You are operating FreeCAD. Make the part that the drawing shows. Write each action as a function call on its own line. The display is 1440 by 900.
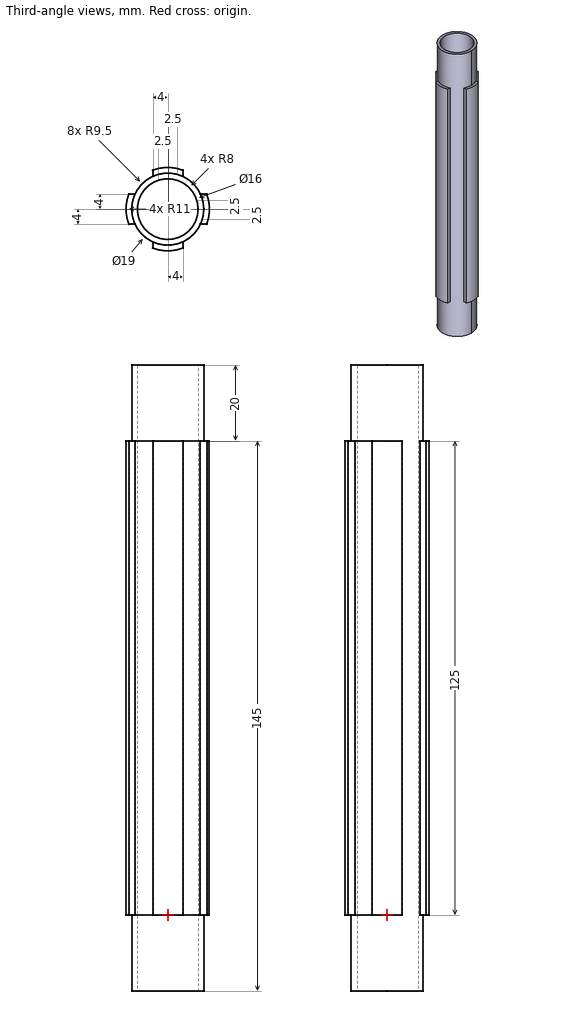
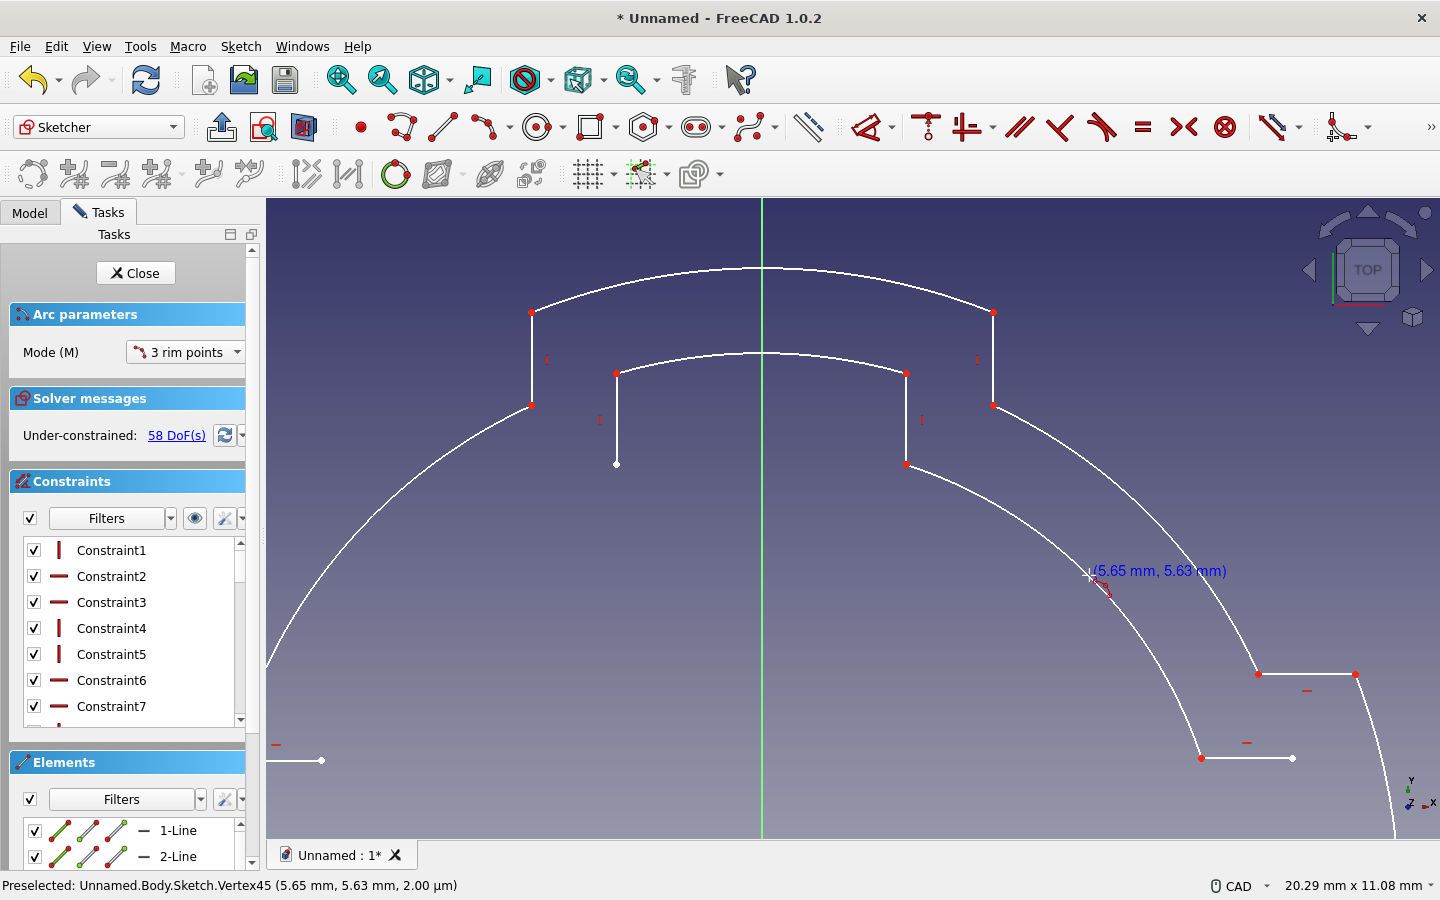
scroll(794, 353, down, 6)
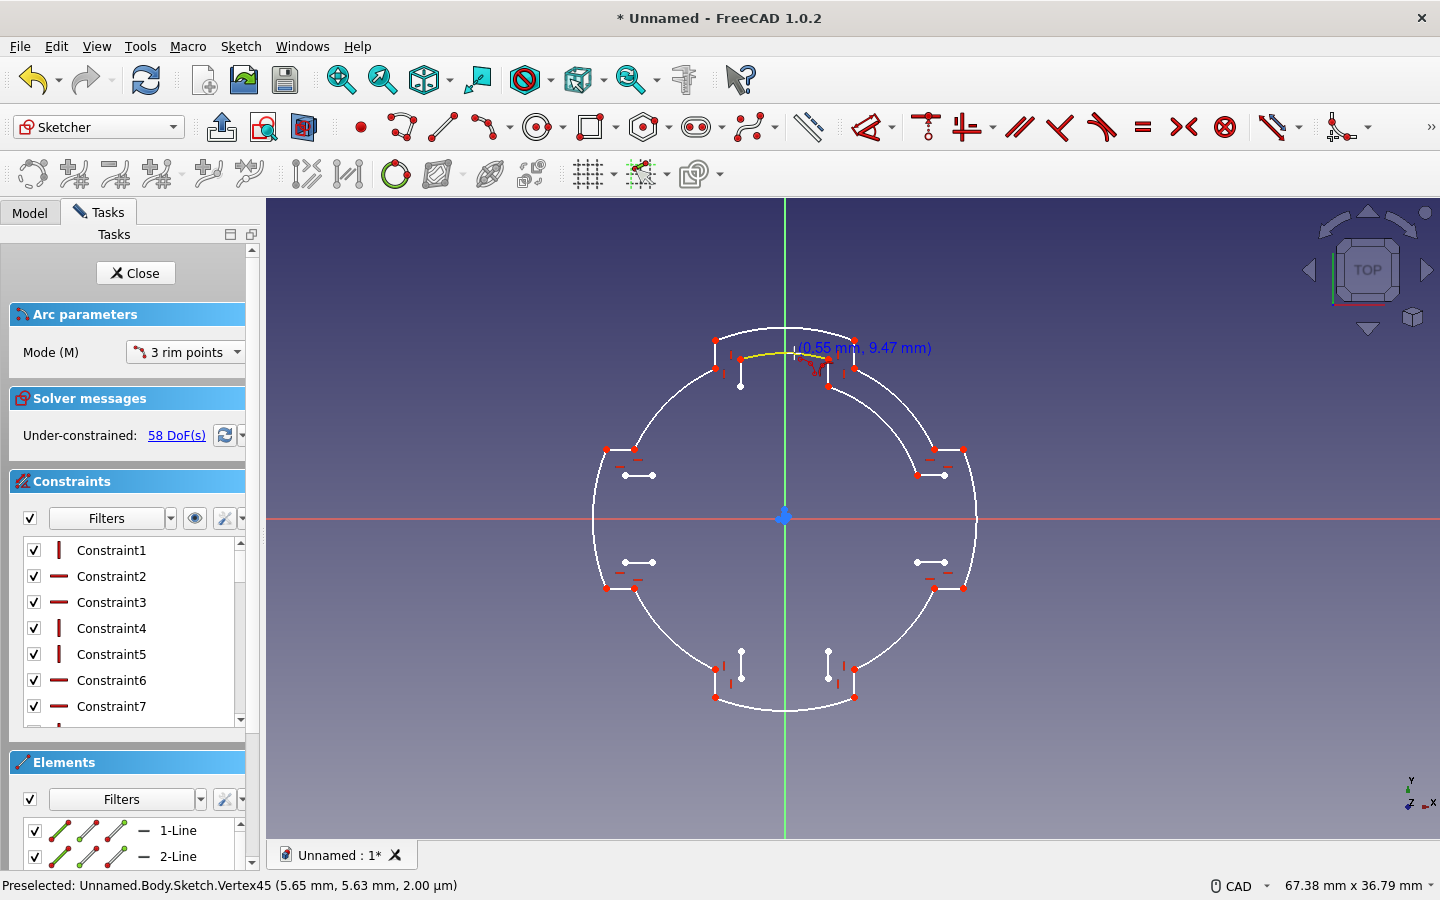
click(945, 475)
click(945, 562)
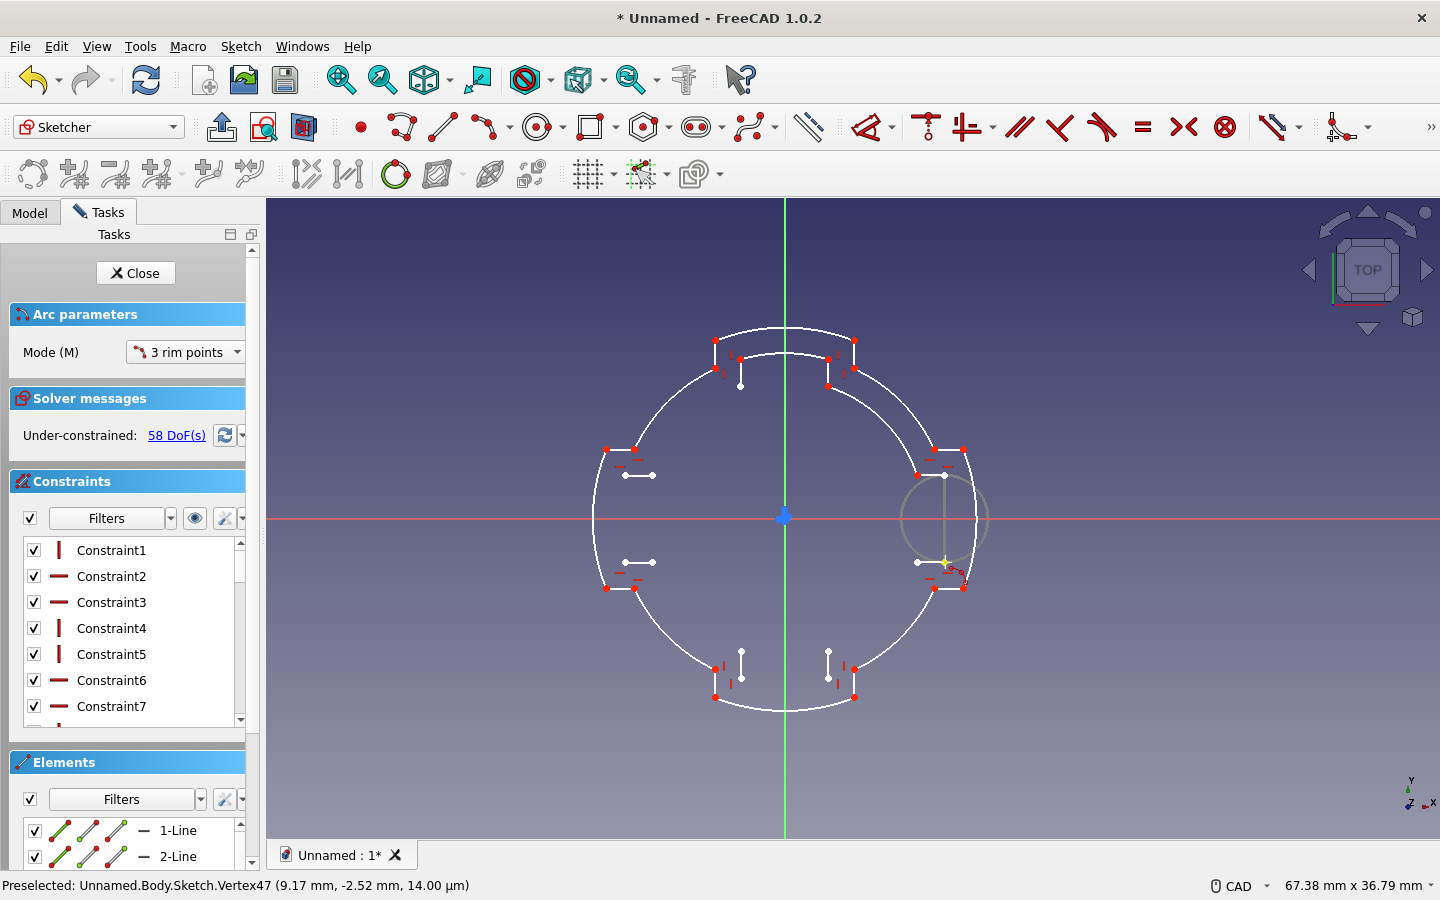
scroll(950, 527, up, 6)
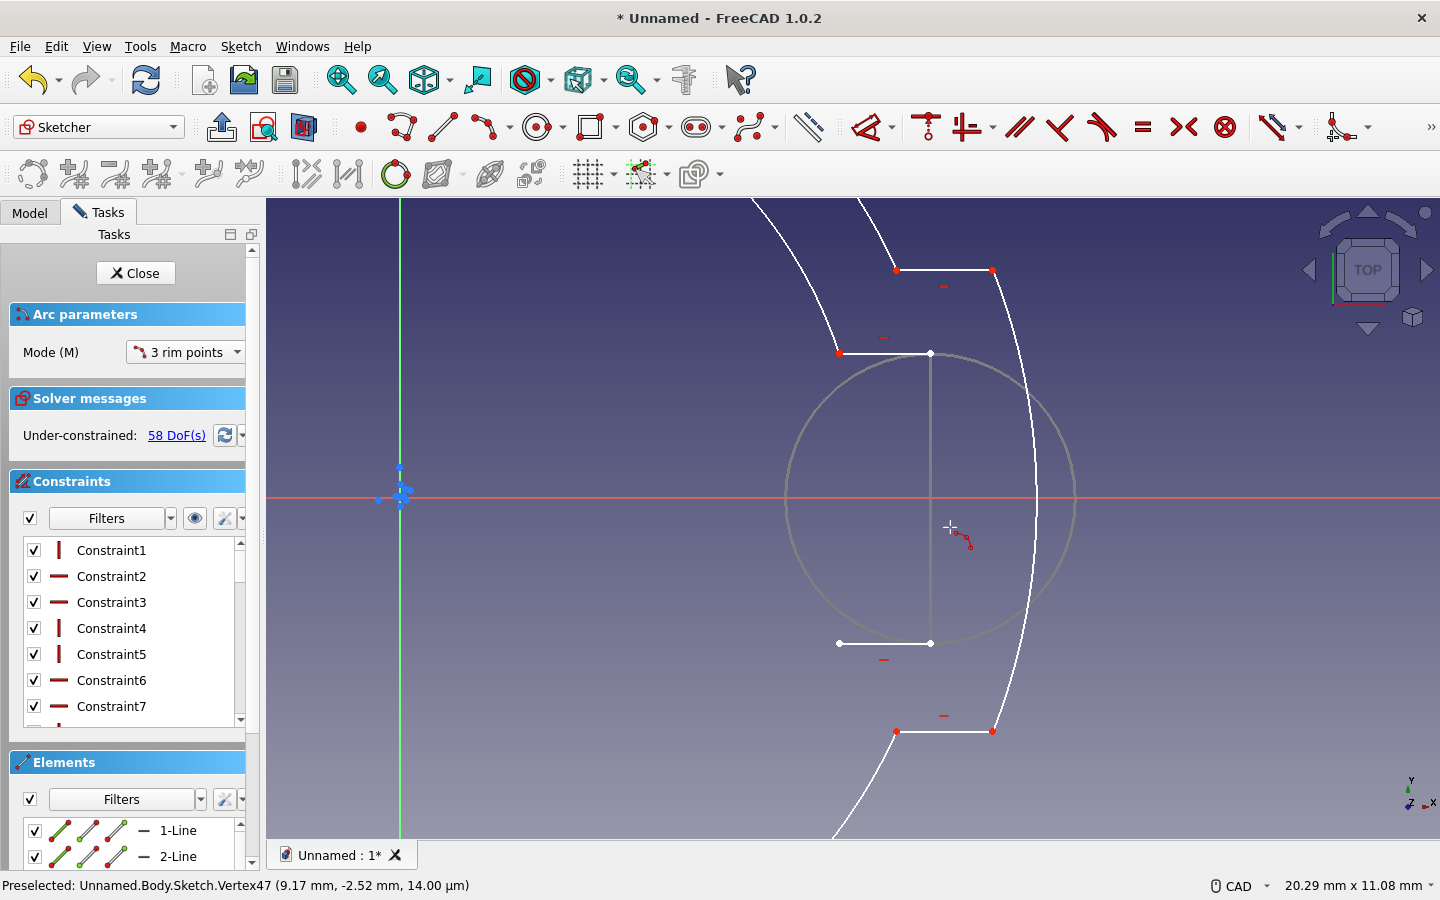
click(949, 527)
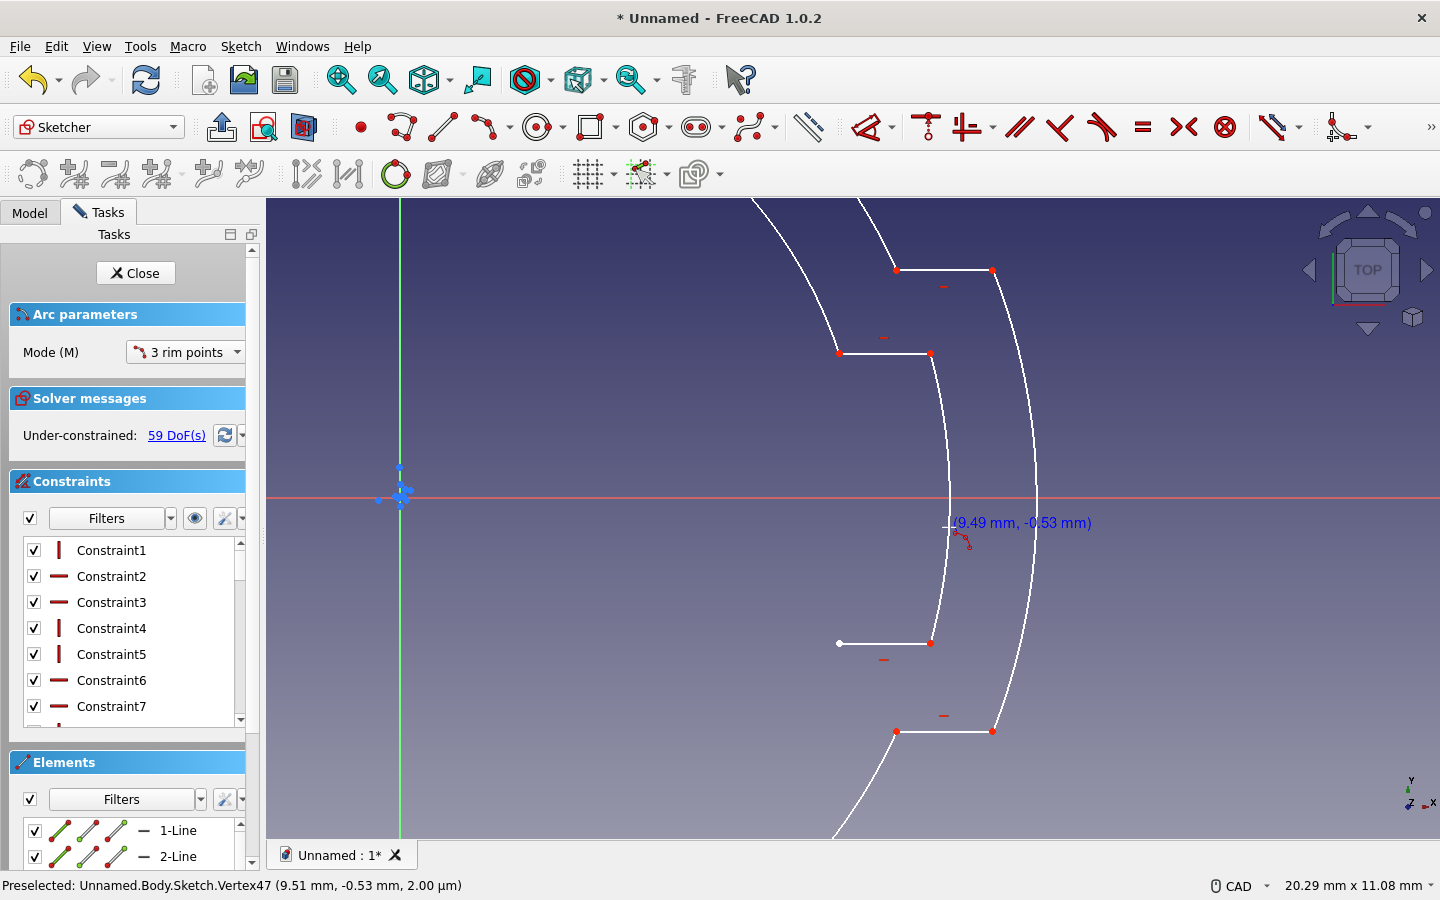
click(839, 644)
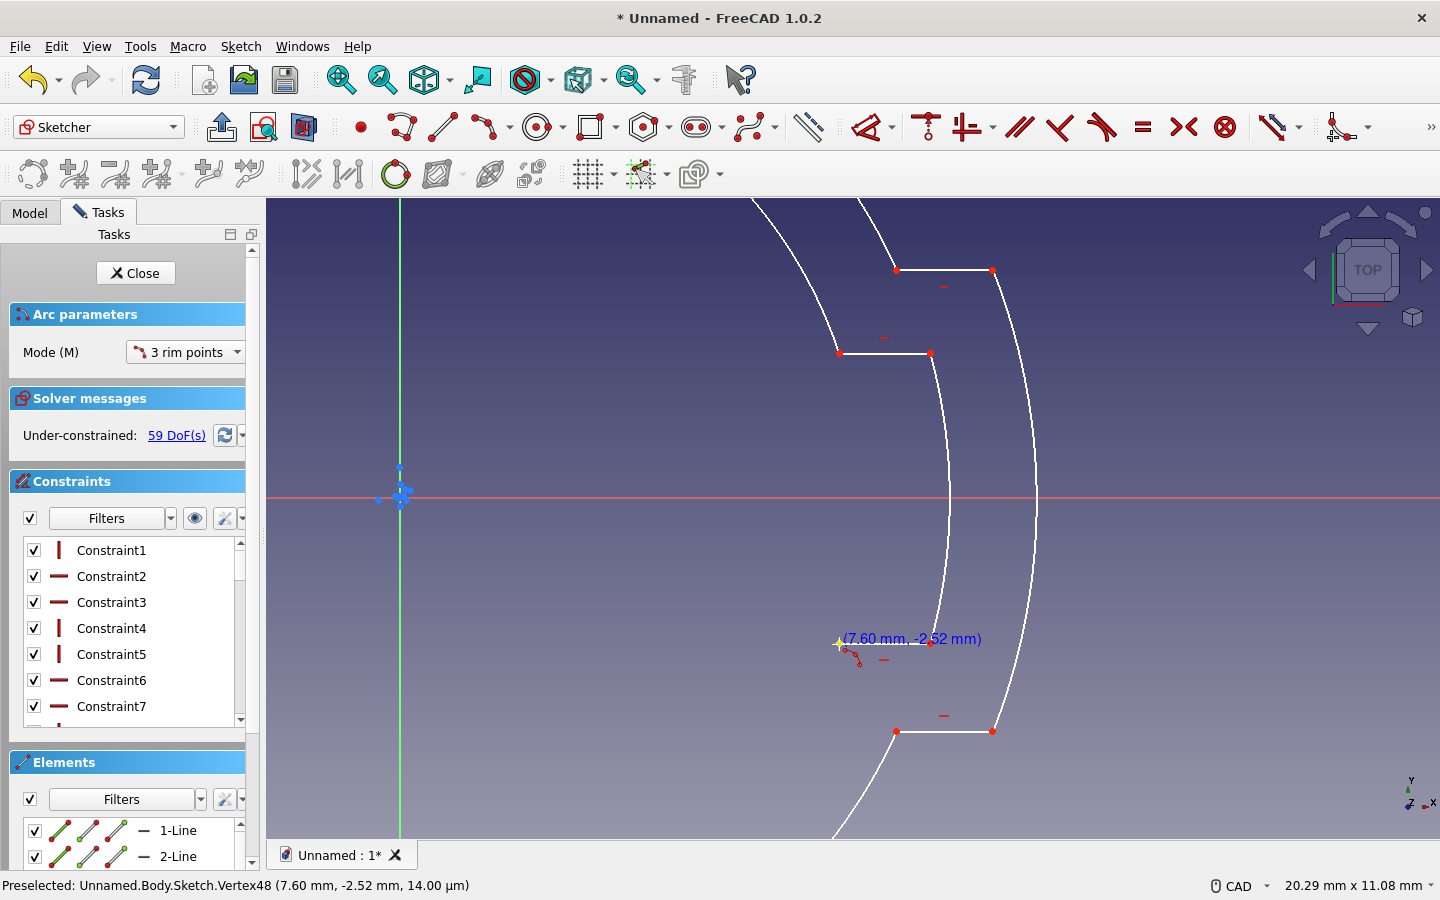
scroll(950, 528, down, 6)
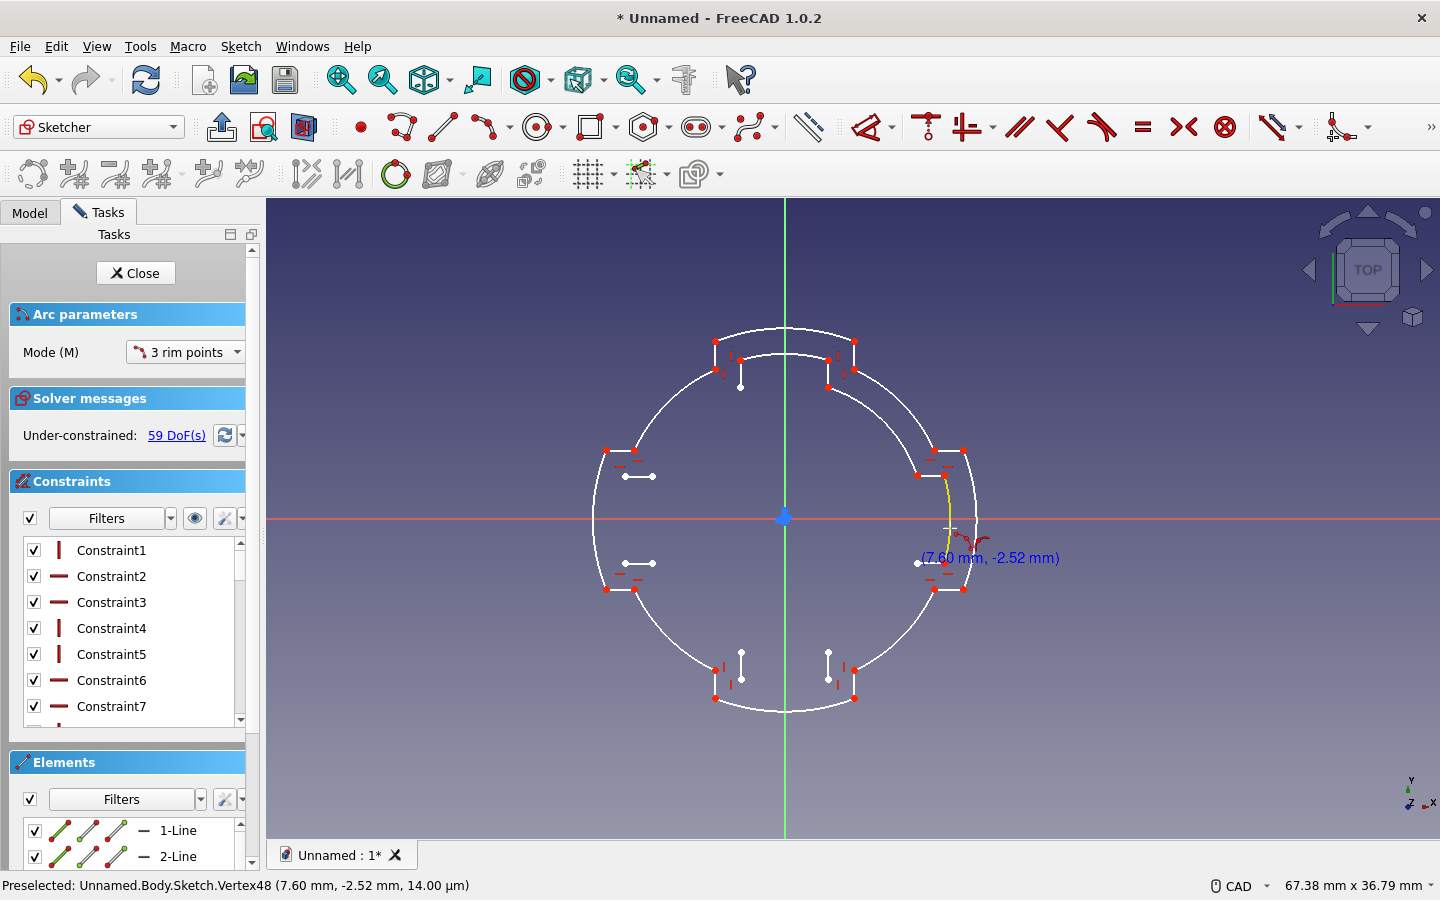
click(828, 653)
click(883, 618)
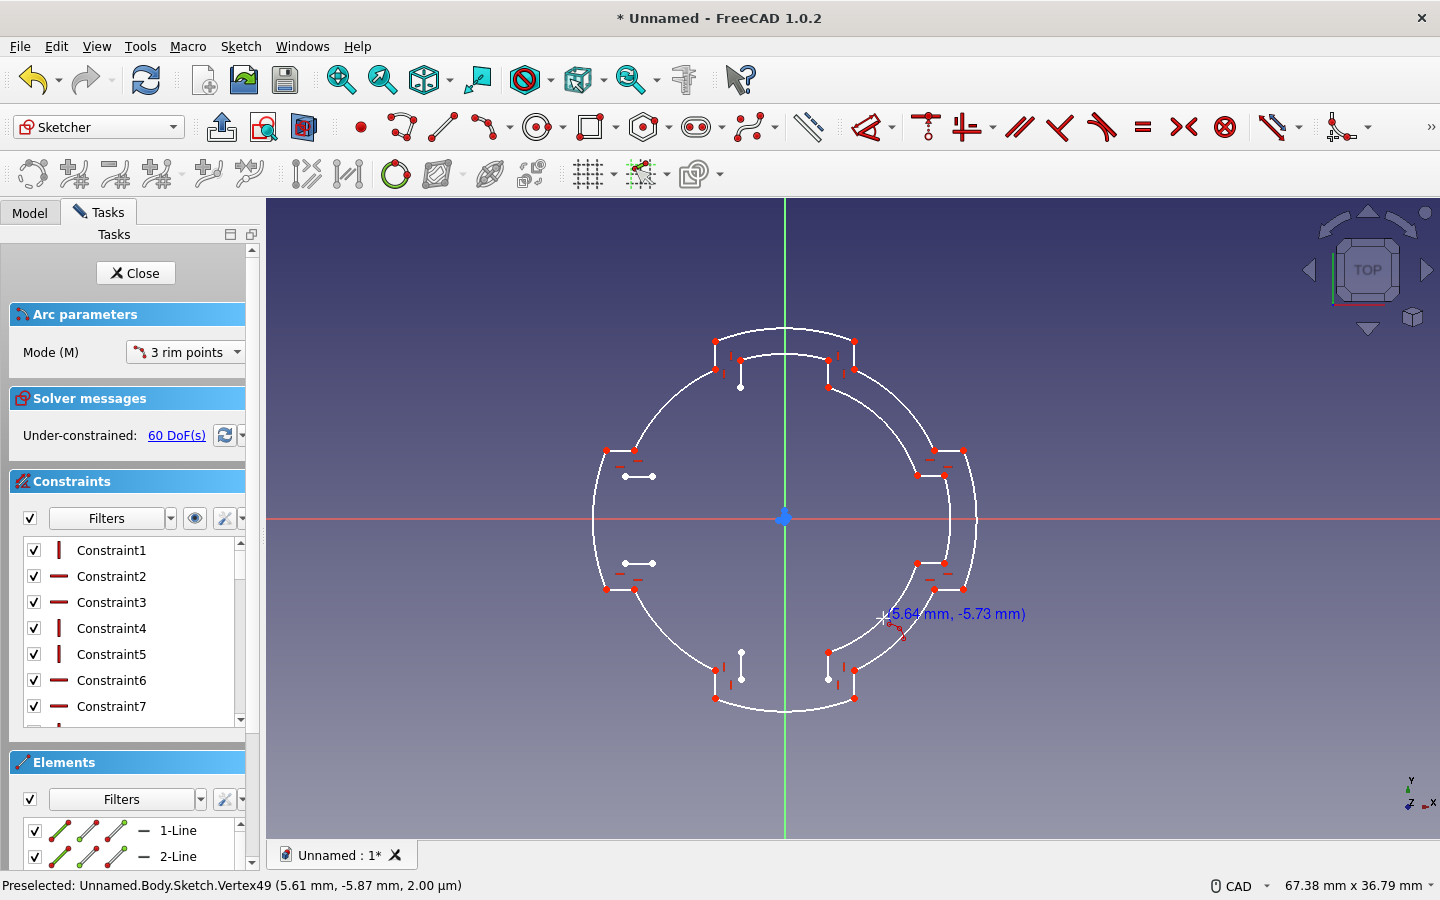
click(828, 680)
click(741, 680)